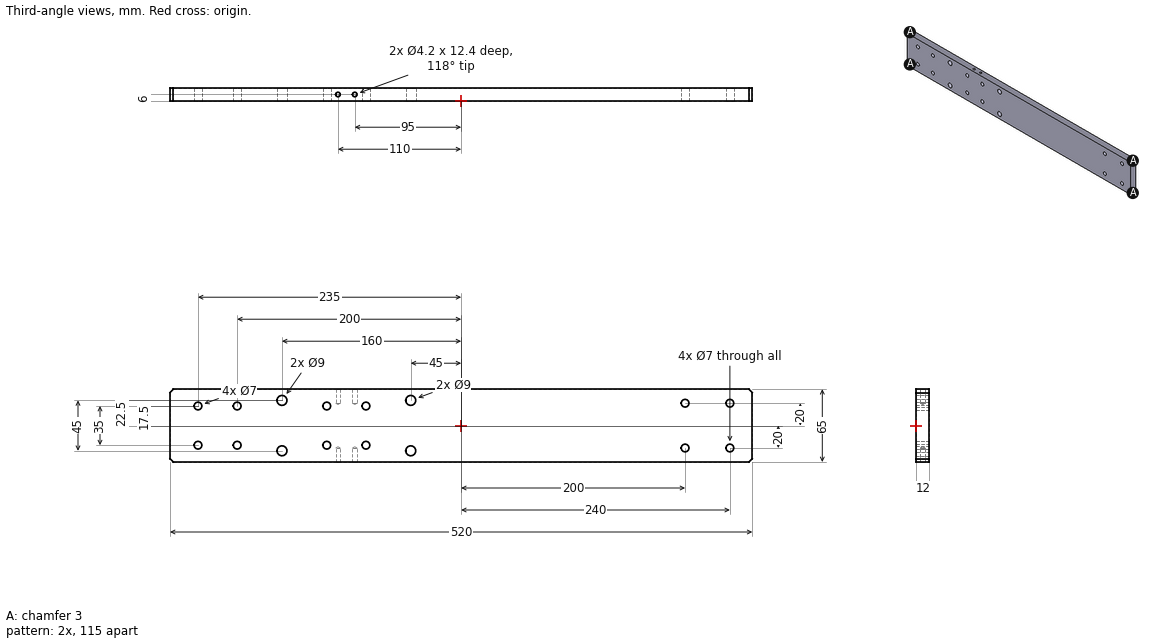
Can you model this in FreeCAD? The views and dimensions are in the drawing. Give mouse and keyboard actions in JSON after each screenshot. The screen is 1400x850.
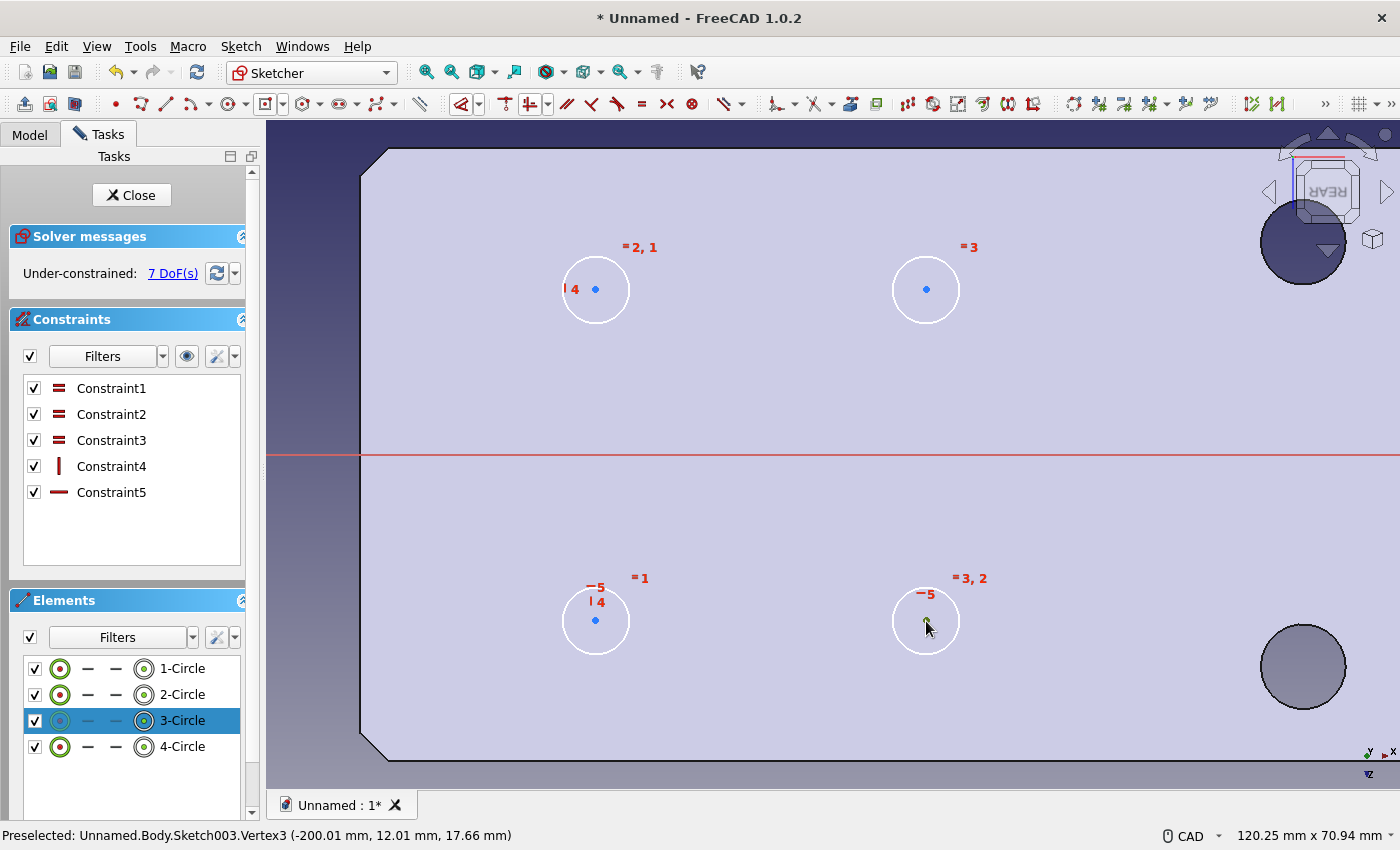
{"action": "left_click", "coordinate": [926, 290]}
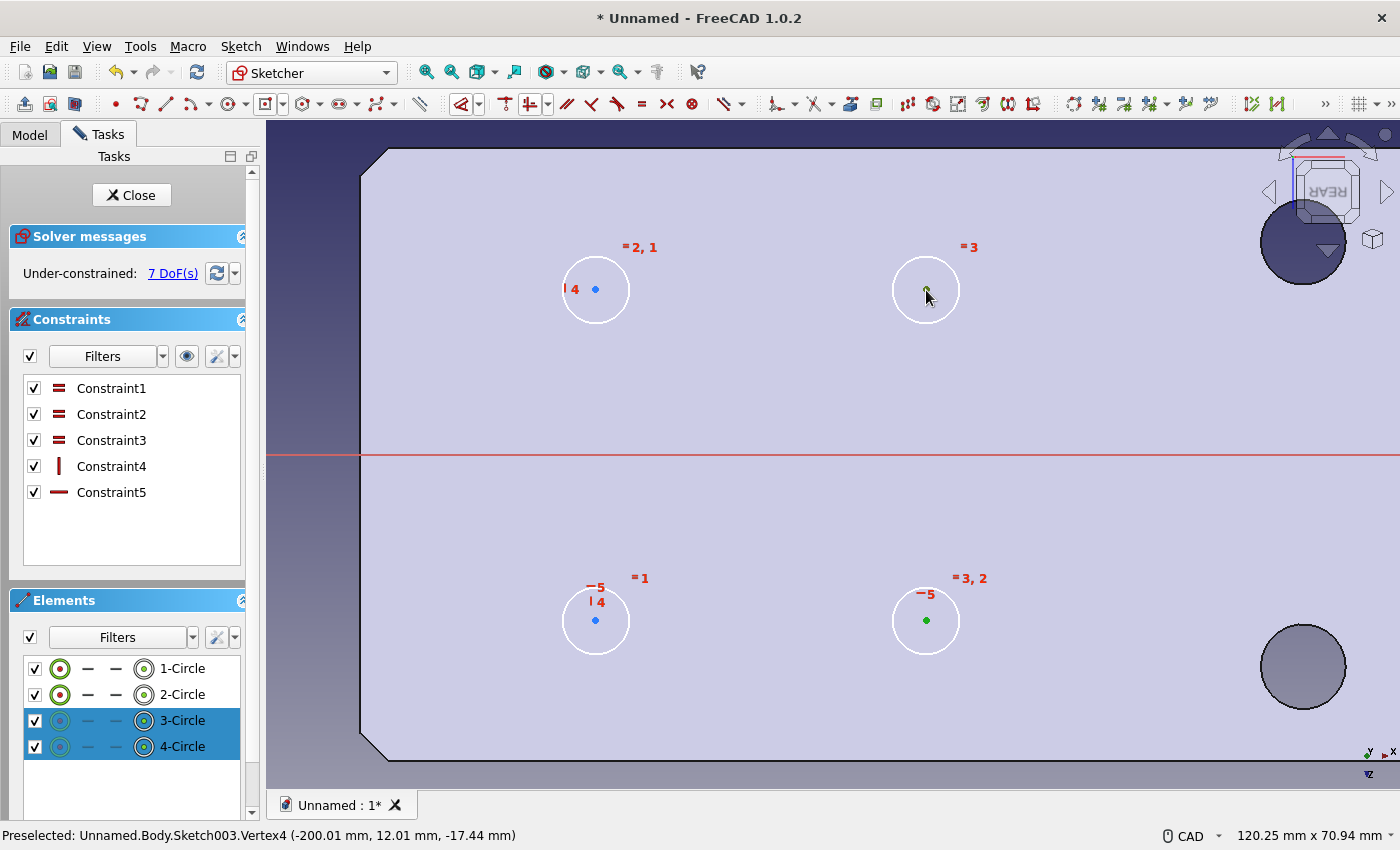
{"action": "left_click", "coordinate": [548, 104]}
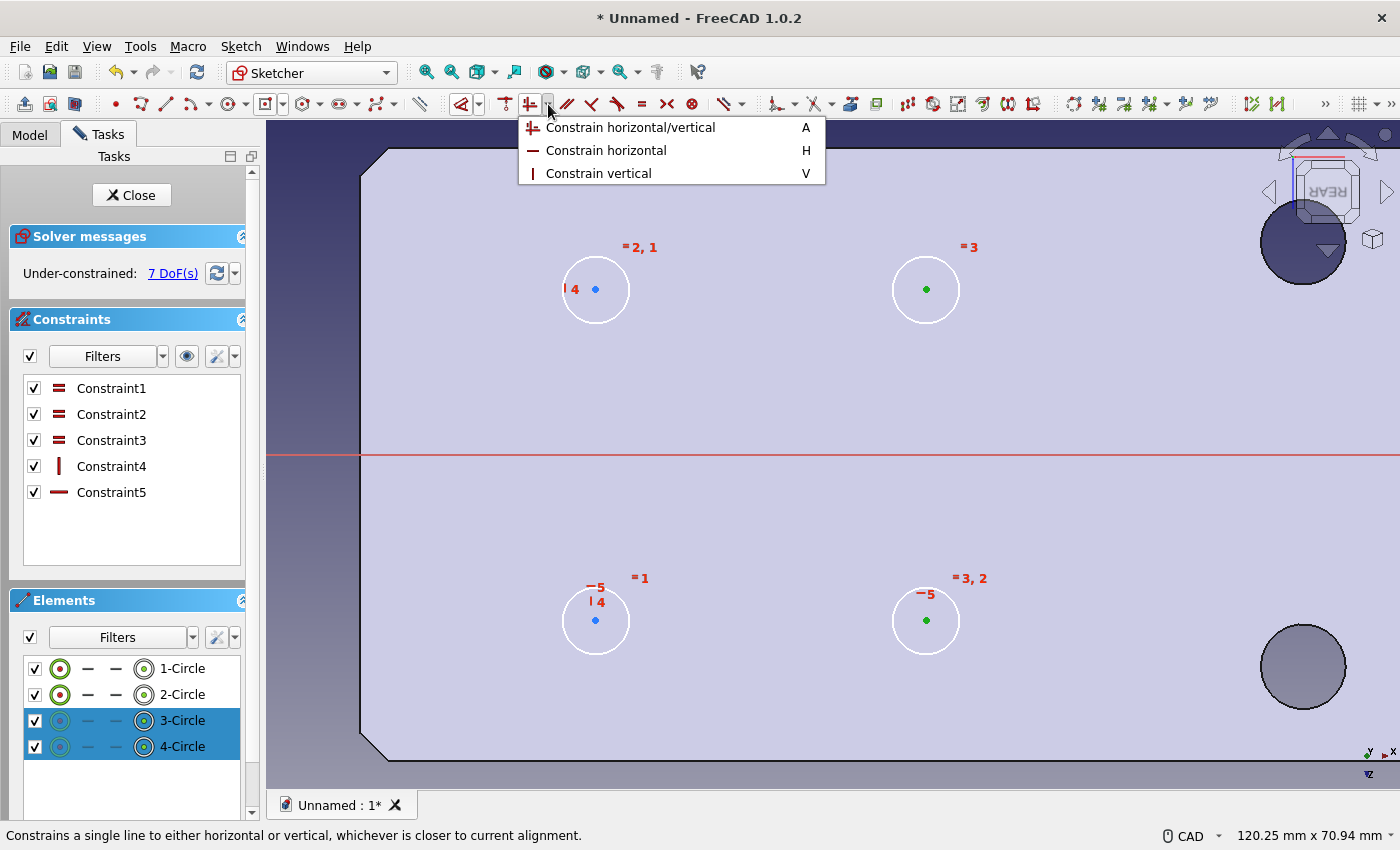
{"action": "left_click", "coordinate": [672, 174]}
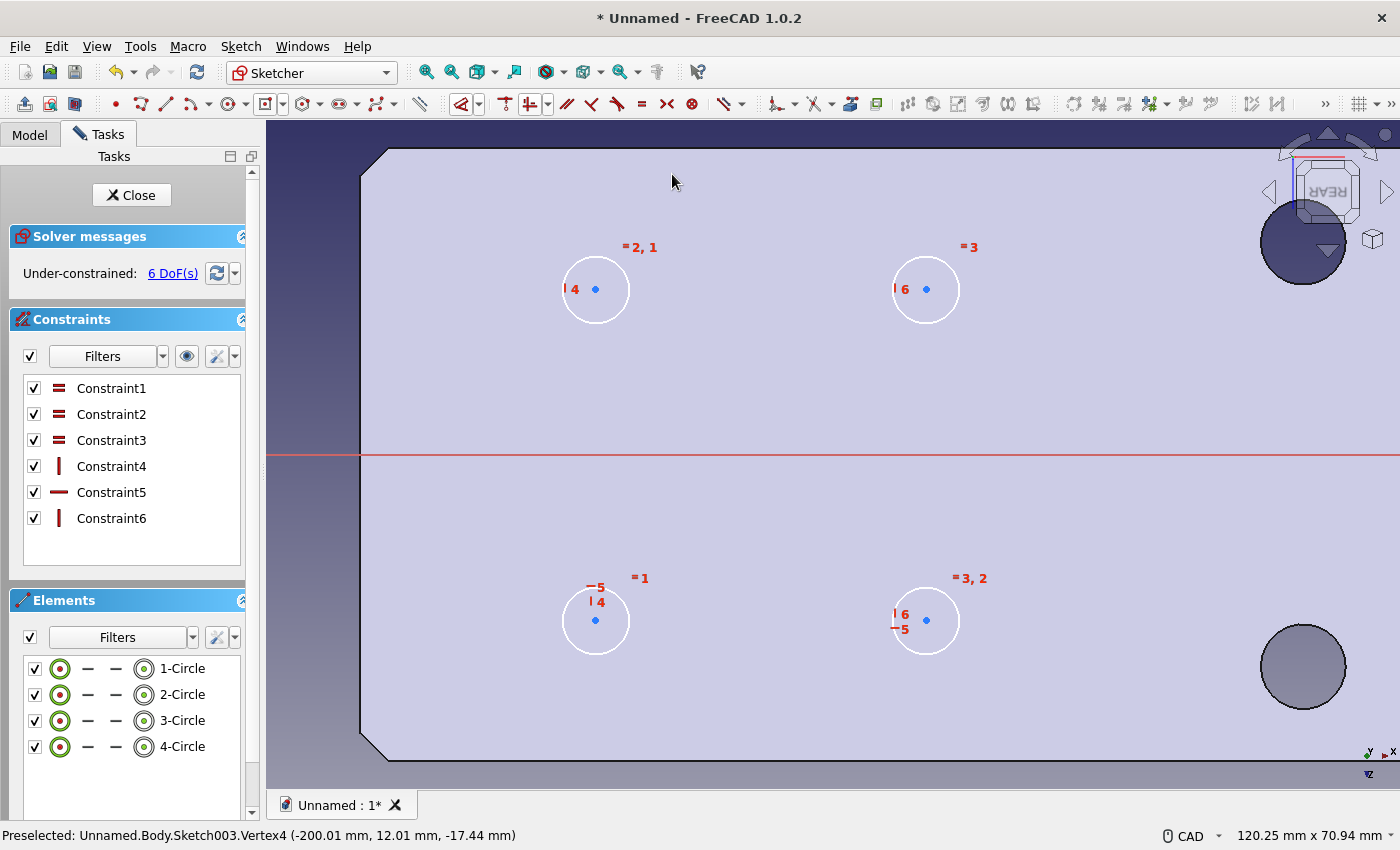
{"action": "left_click", "coordinate": [596, 290]}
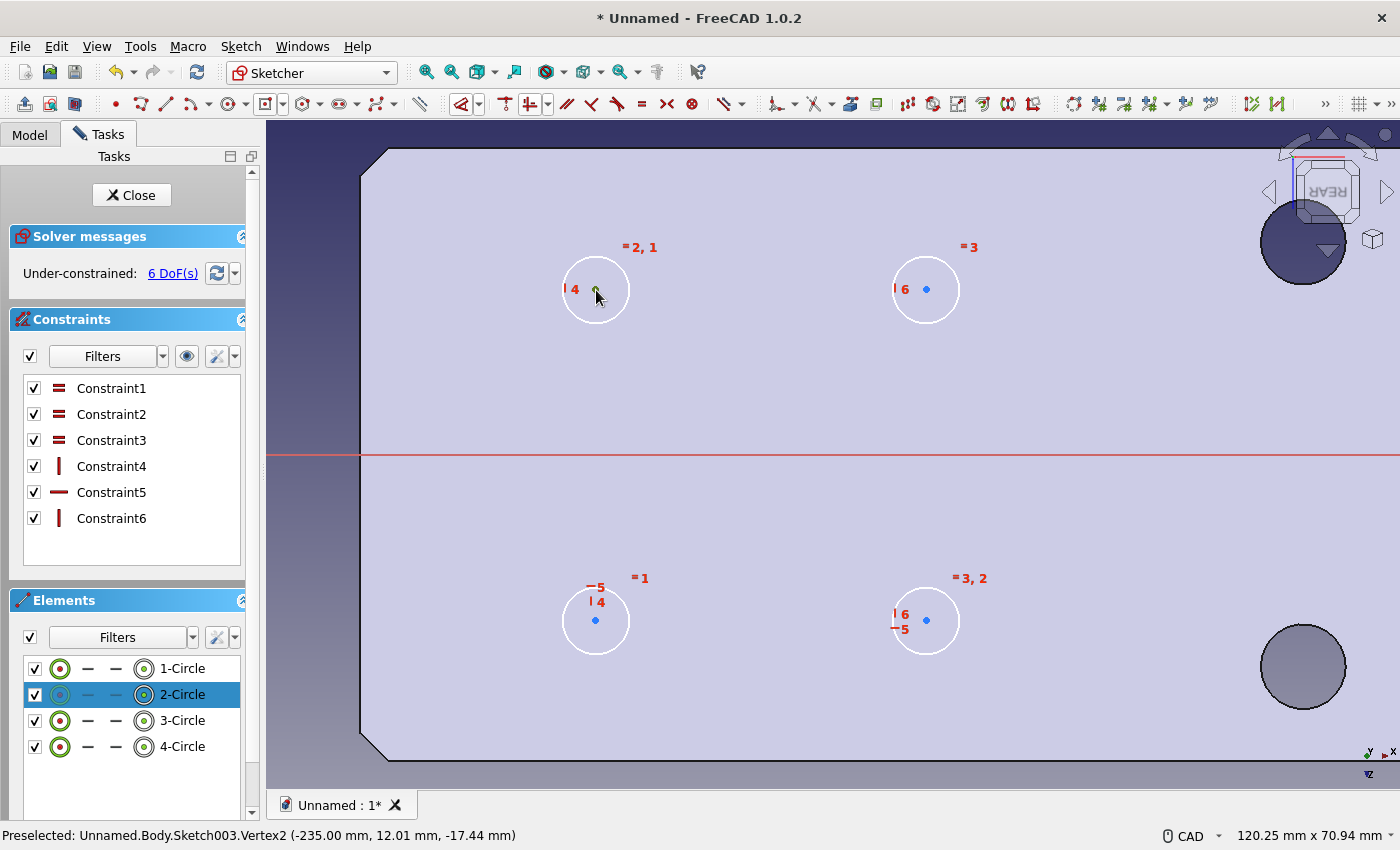
{"action": "left_click", "coordinate": [926, 290]}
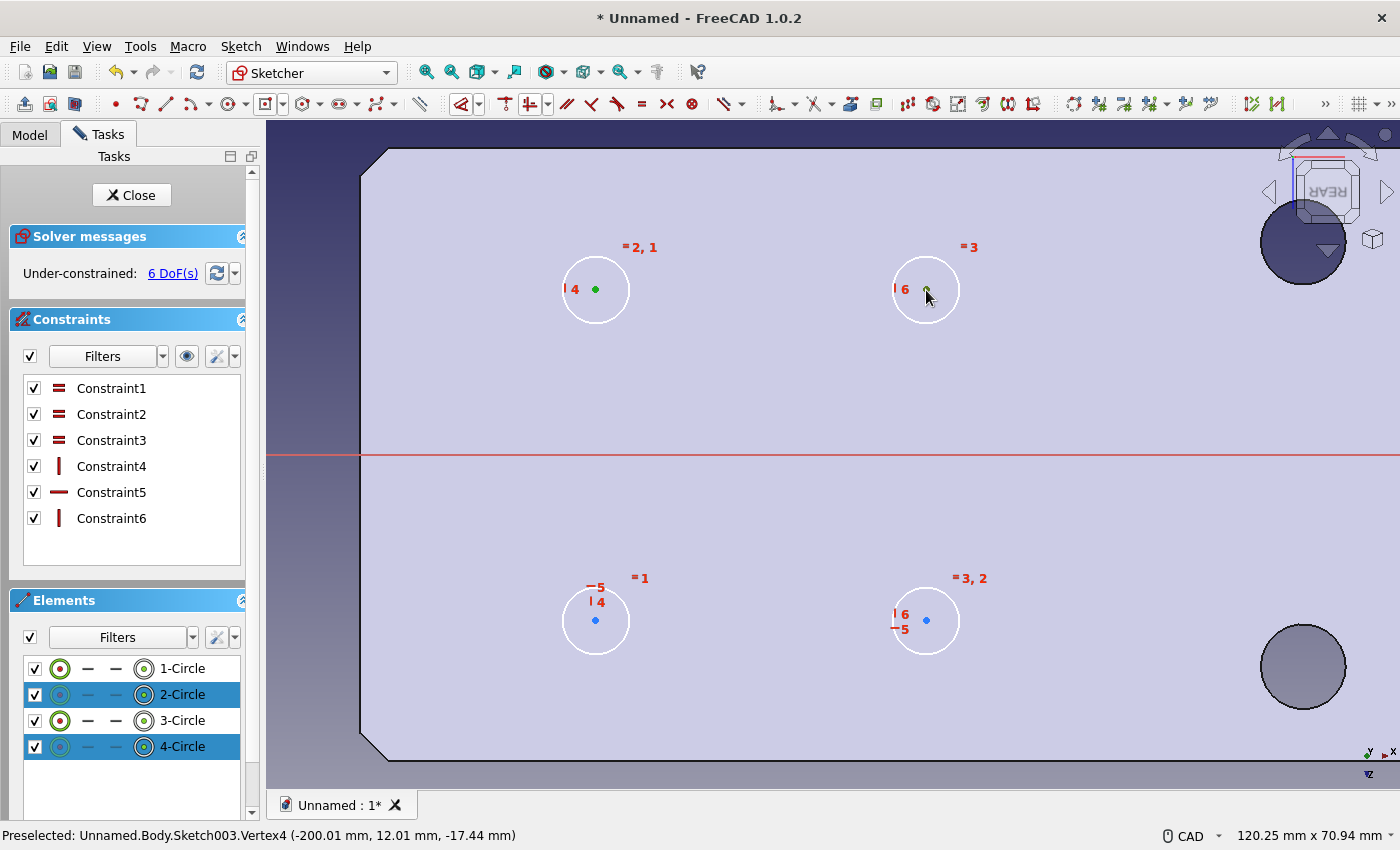
{"action": "key", "text": "h"}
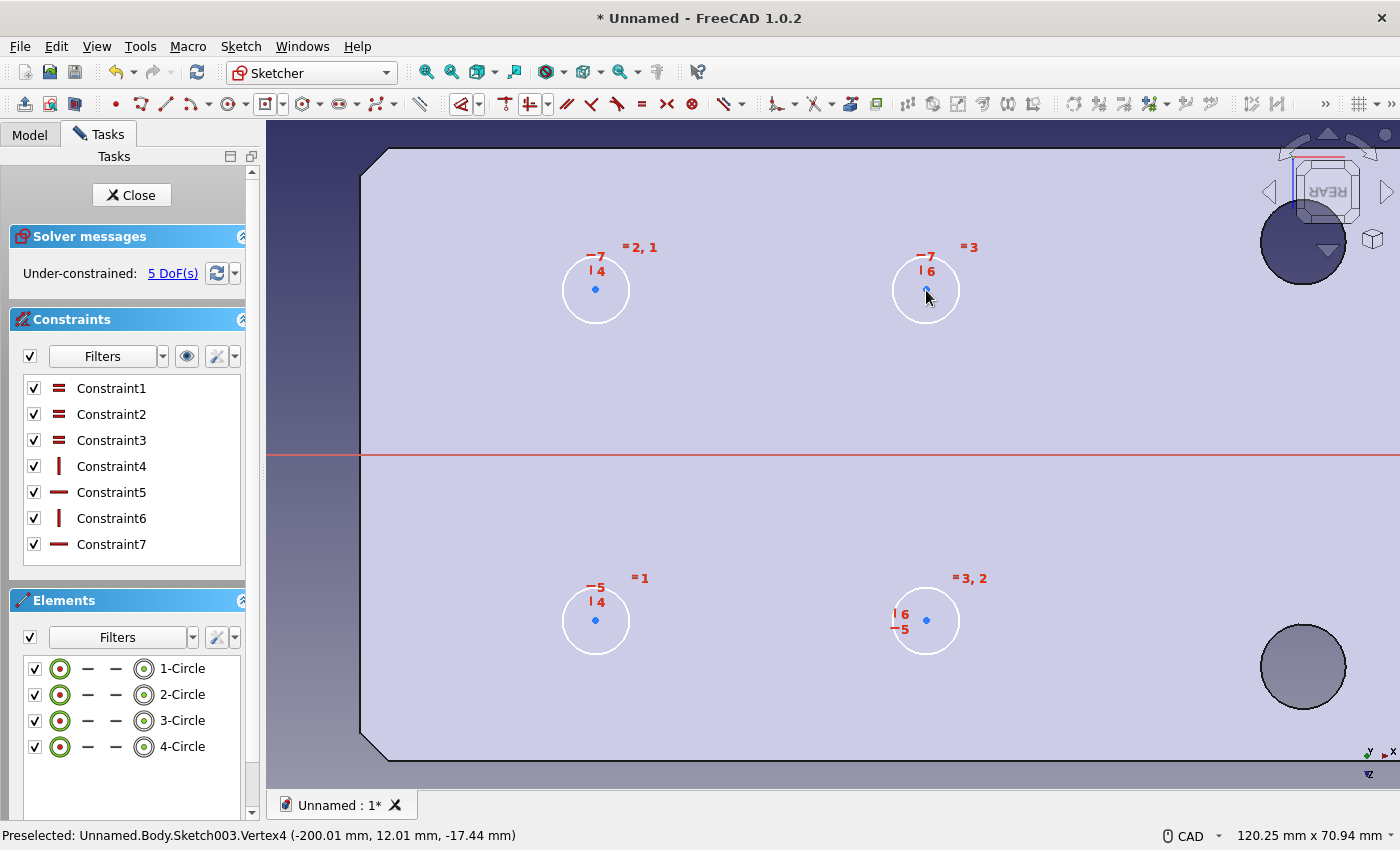
{"action": "left_click", "coordinate": [619, 597]}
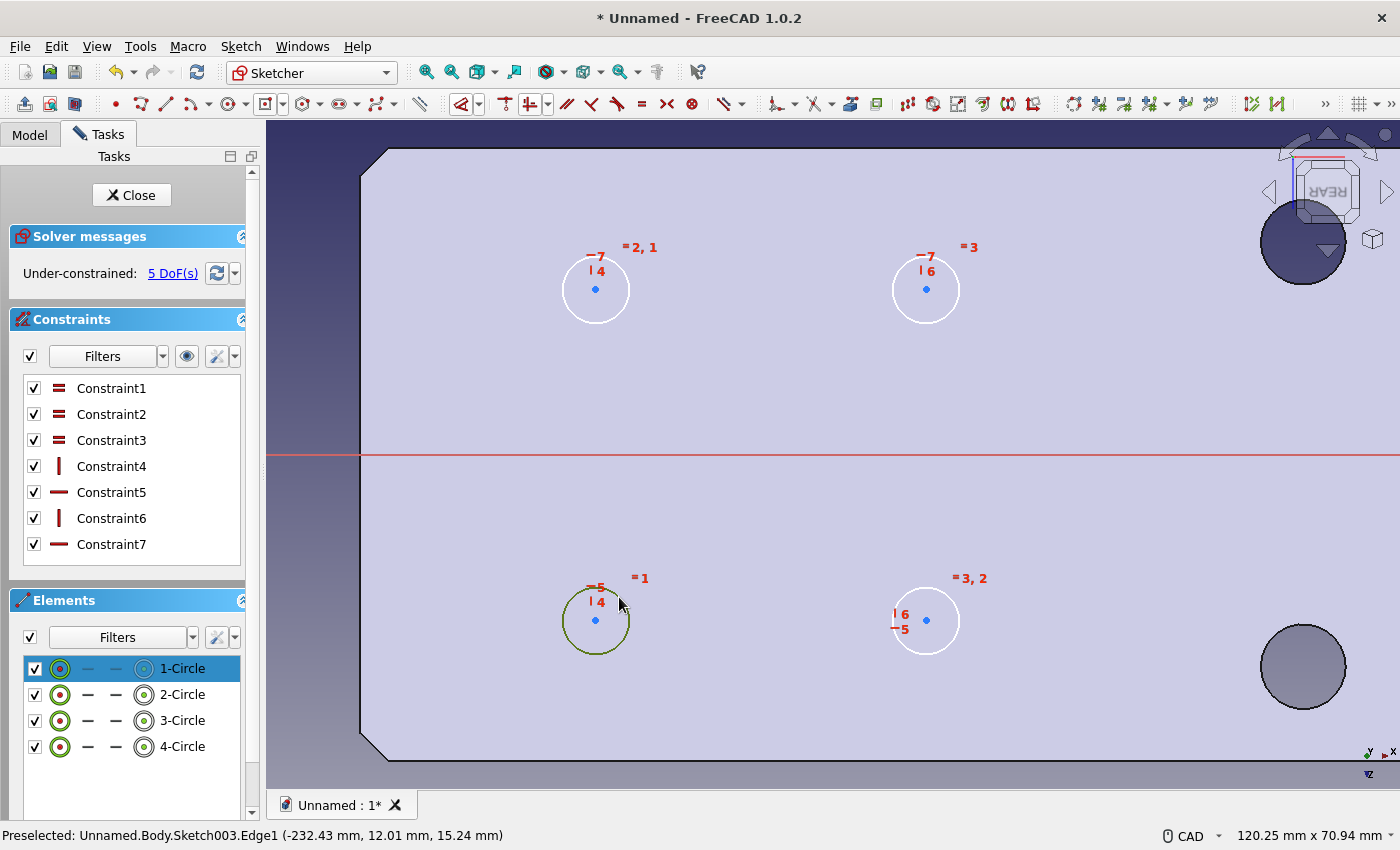
{"action": "left_click", "coordinate": [478, 104]}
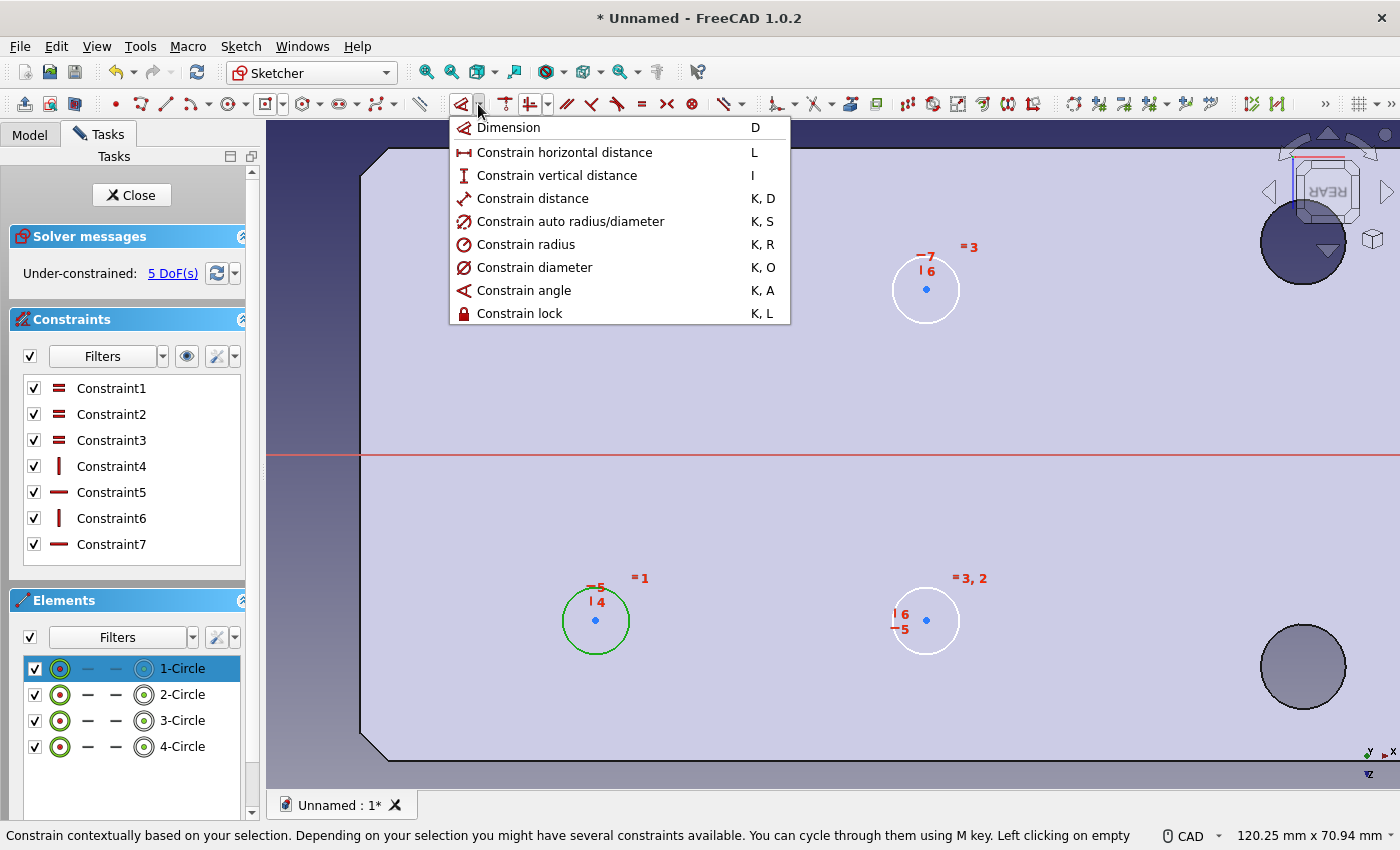
{"action": "left_click", "coordinate": [620, 268]}